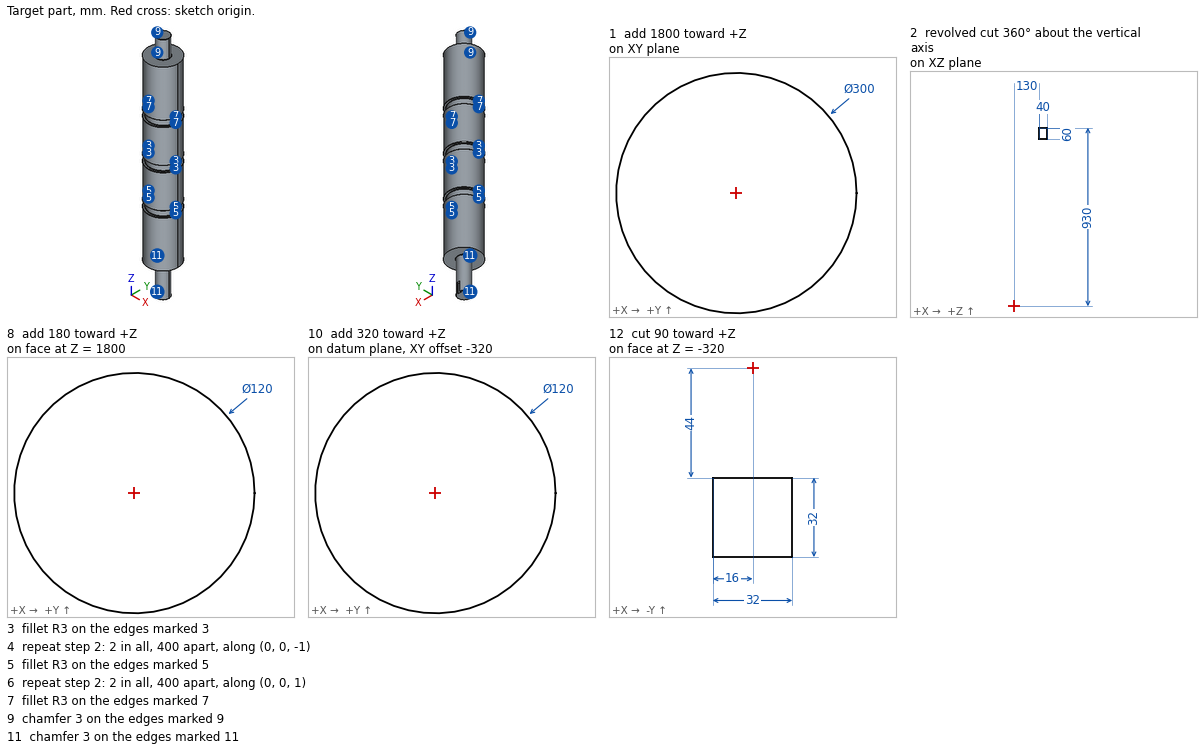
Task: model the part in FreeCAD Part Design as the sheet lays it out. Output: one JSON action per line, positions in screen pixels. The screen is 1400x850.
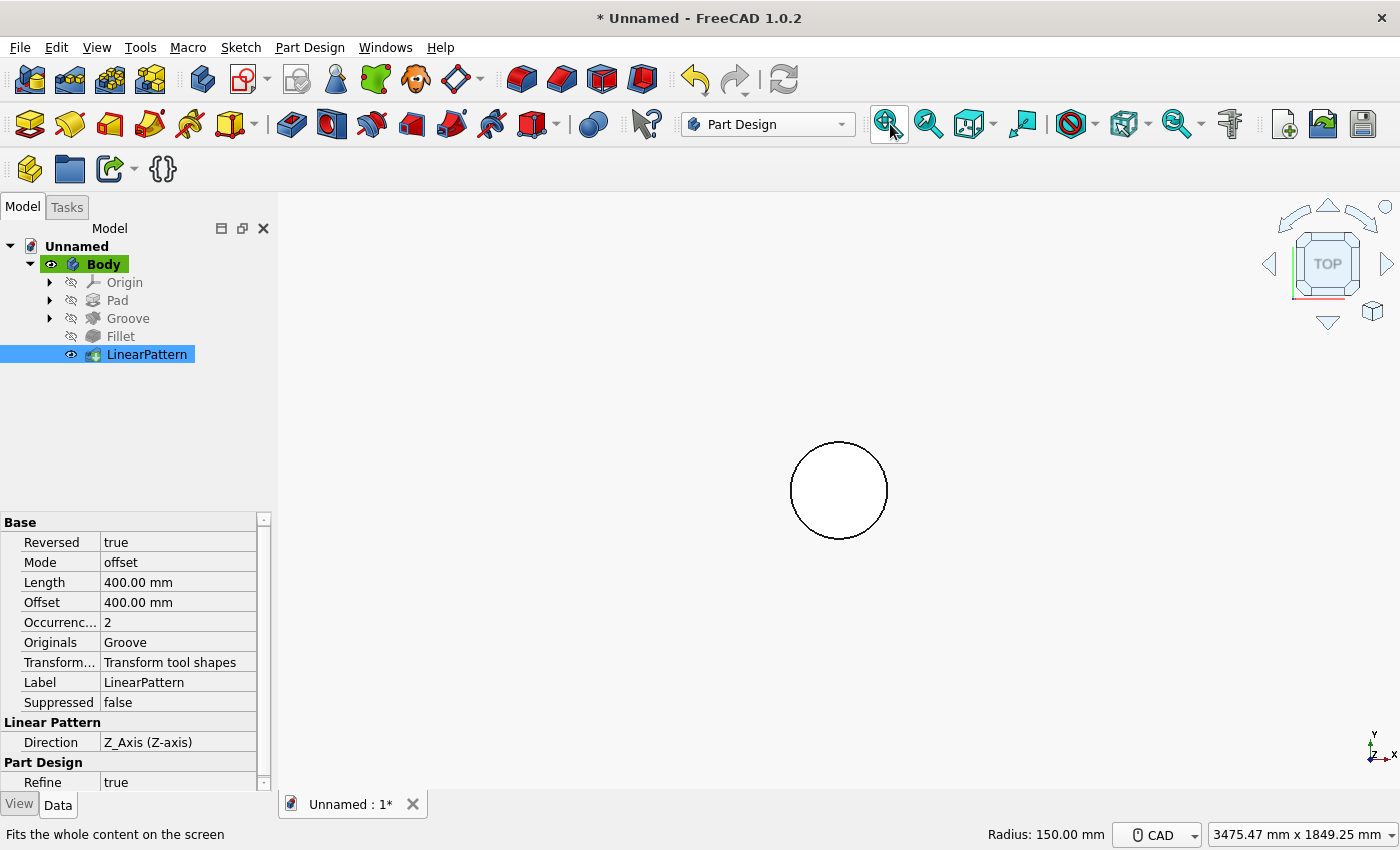
{"action": "key", "text": "0"}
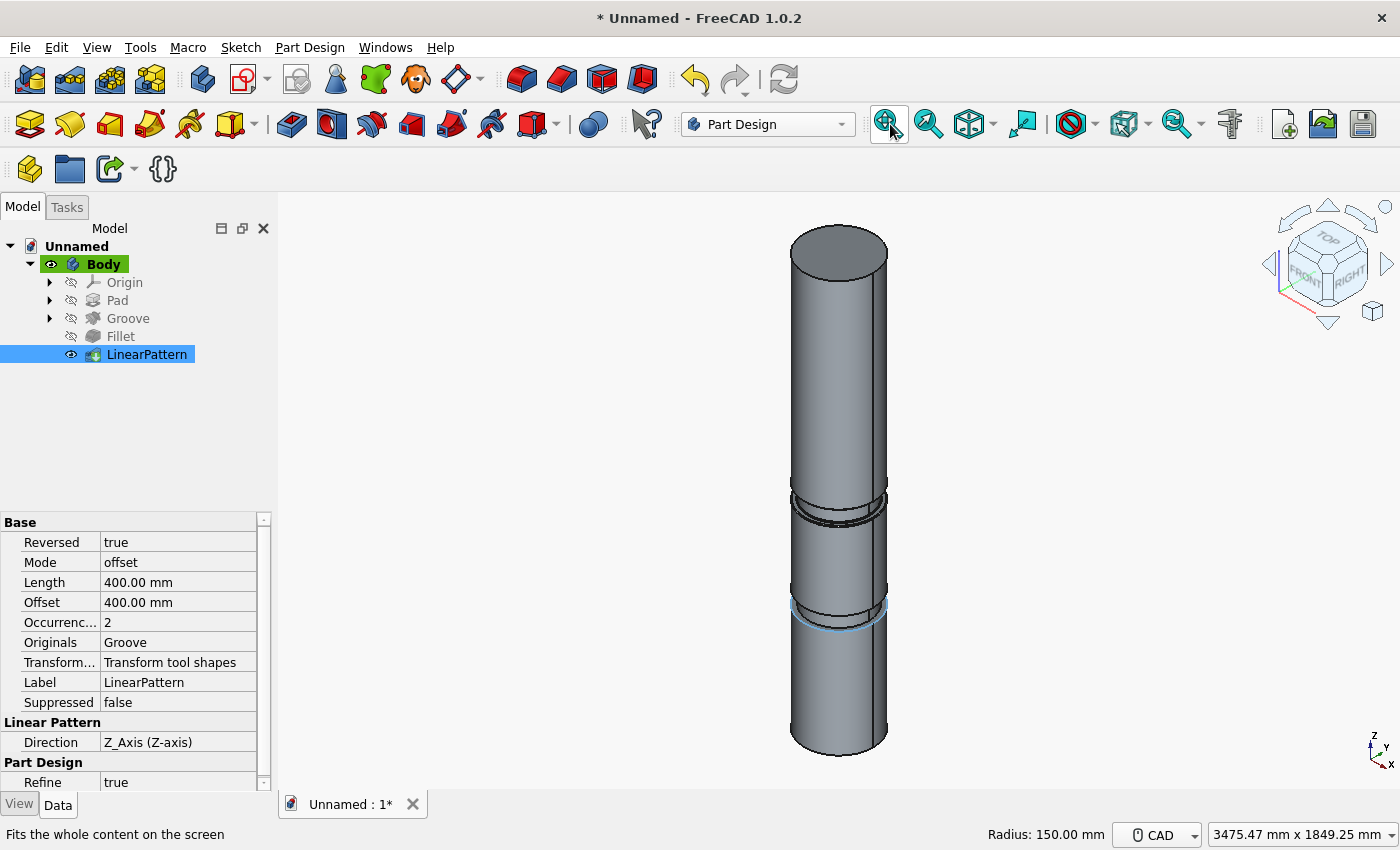
{"action": "key", "text": "1"}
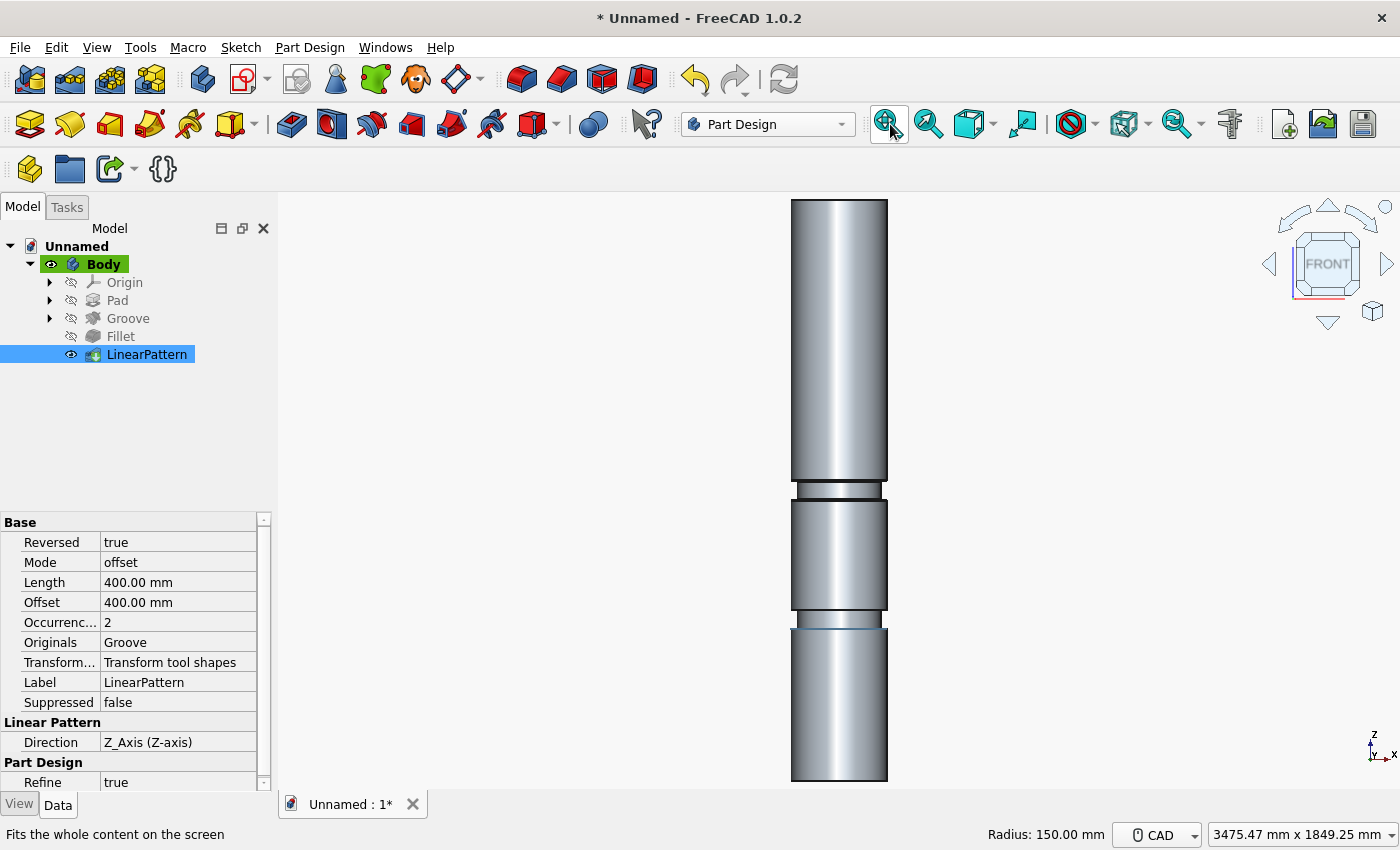
{"action": "left_click", "coordinate": [791, 609], "text": "ctrl"}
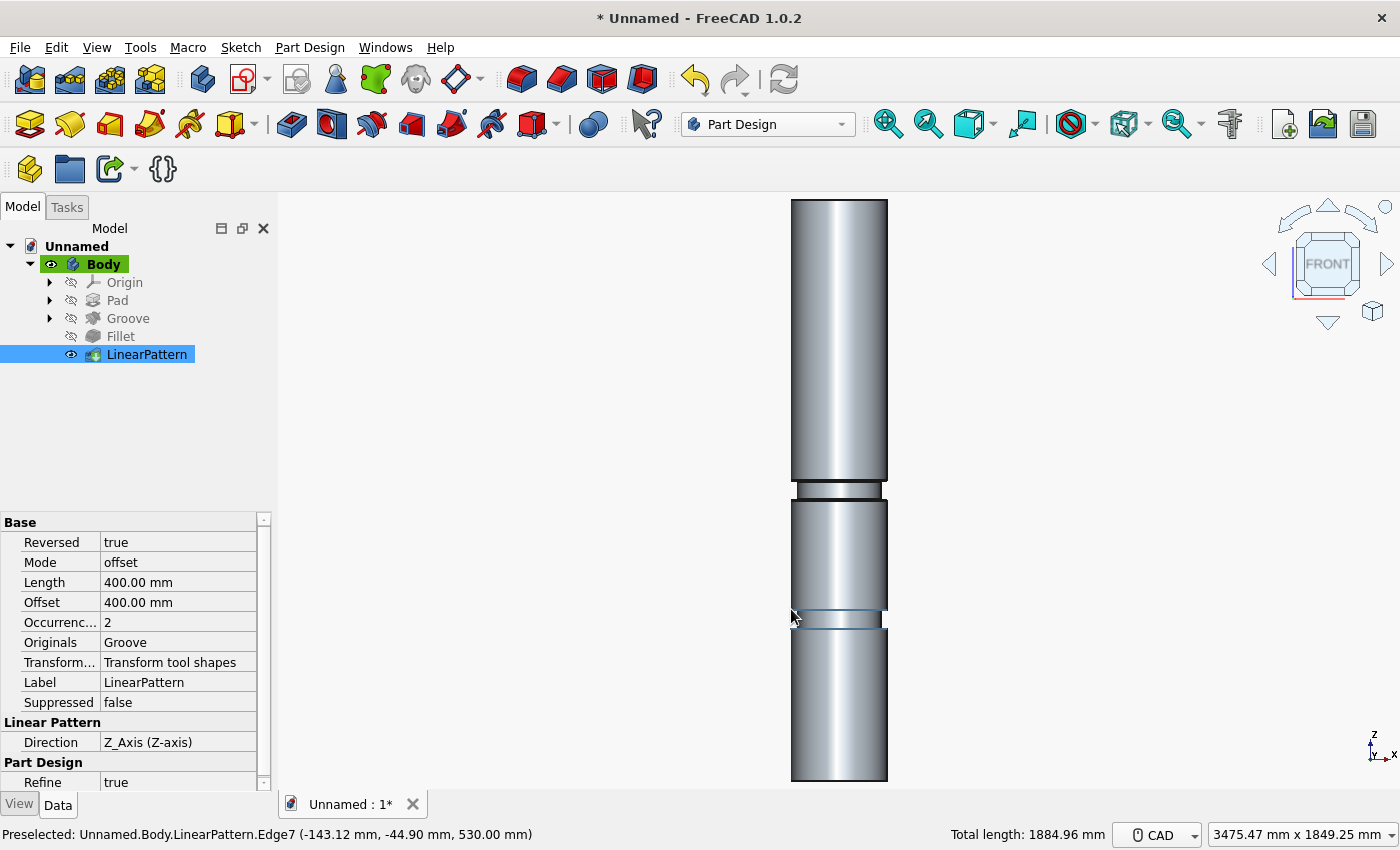
{"action": "key", "text": "3"}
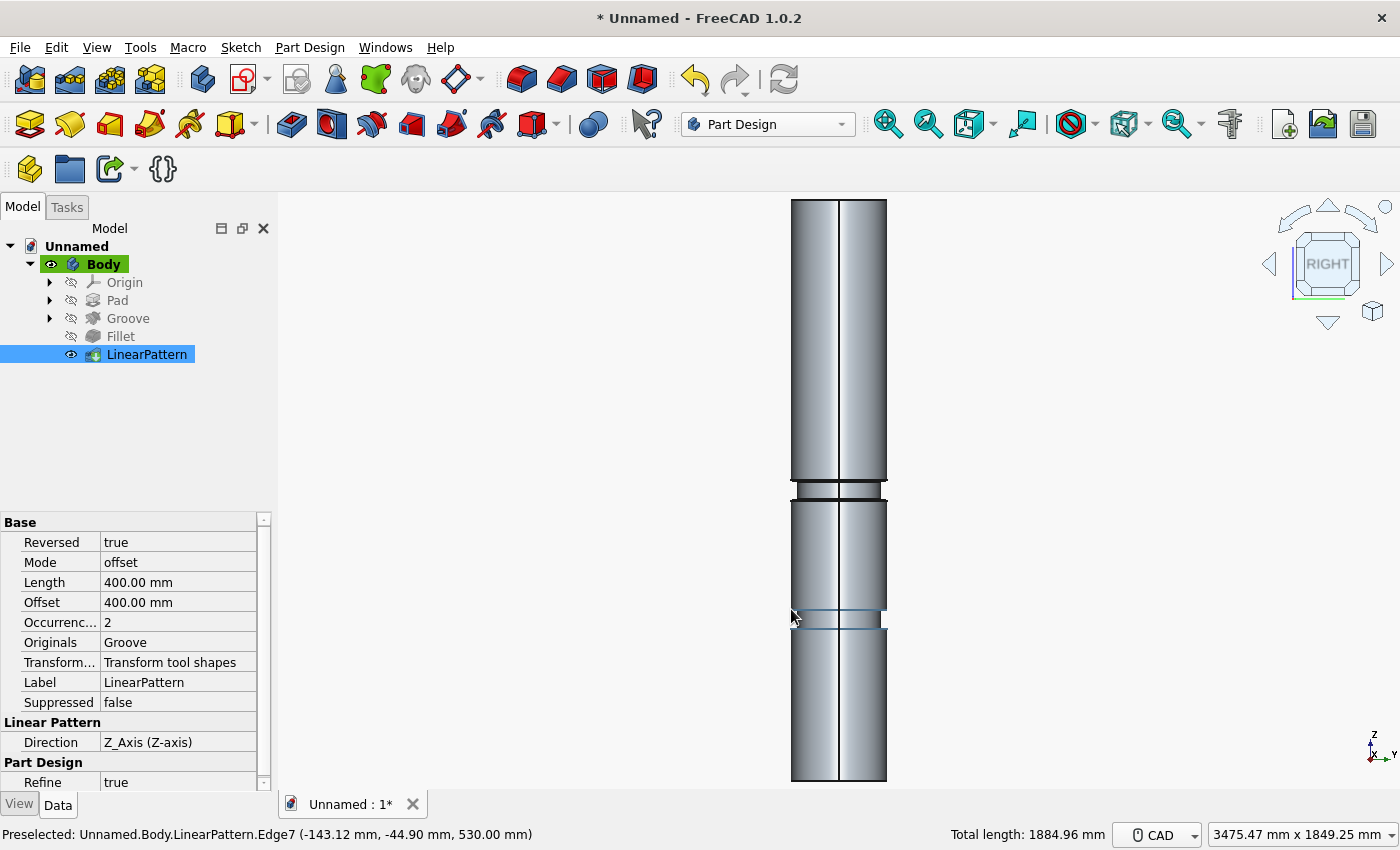
{"action": "key", "text": "5"}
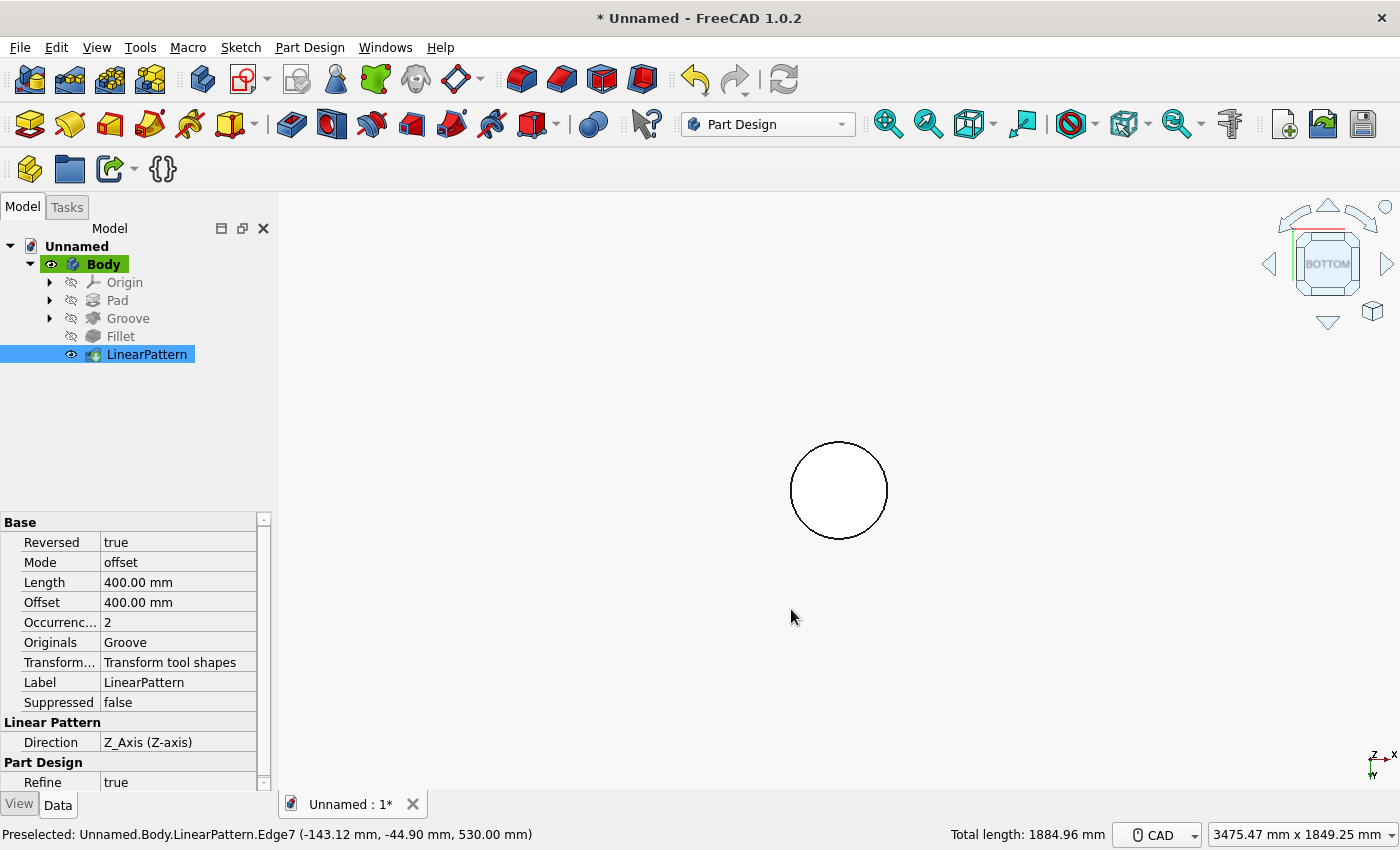
{"action": "left_click", "coordinate": [890, 124]}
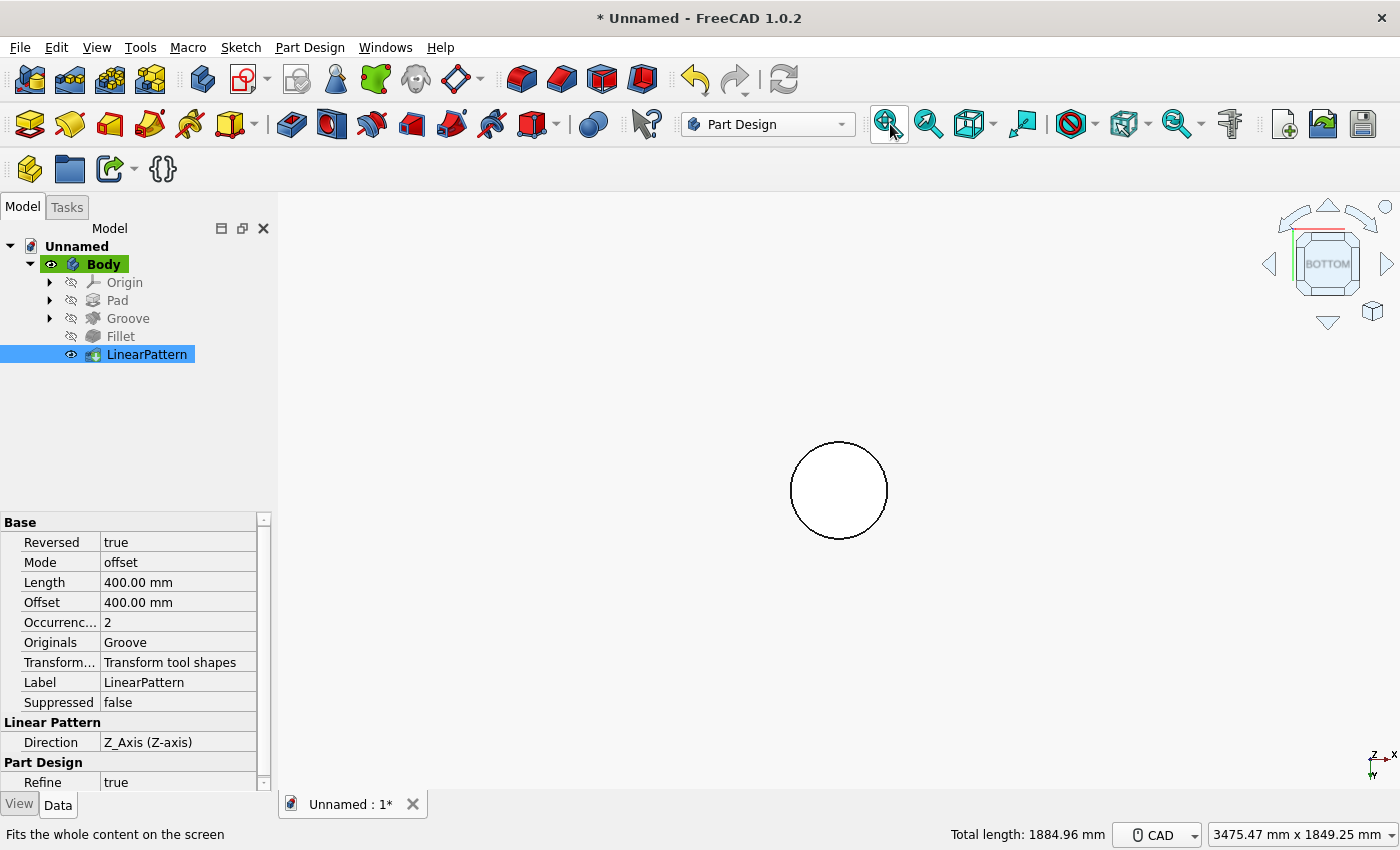
{"action": "key", "text": "4"}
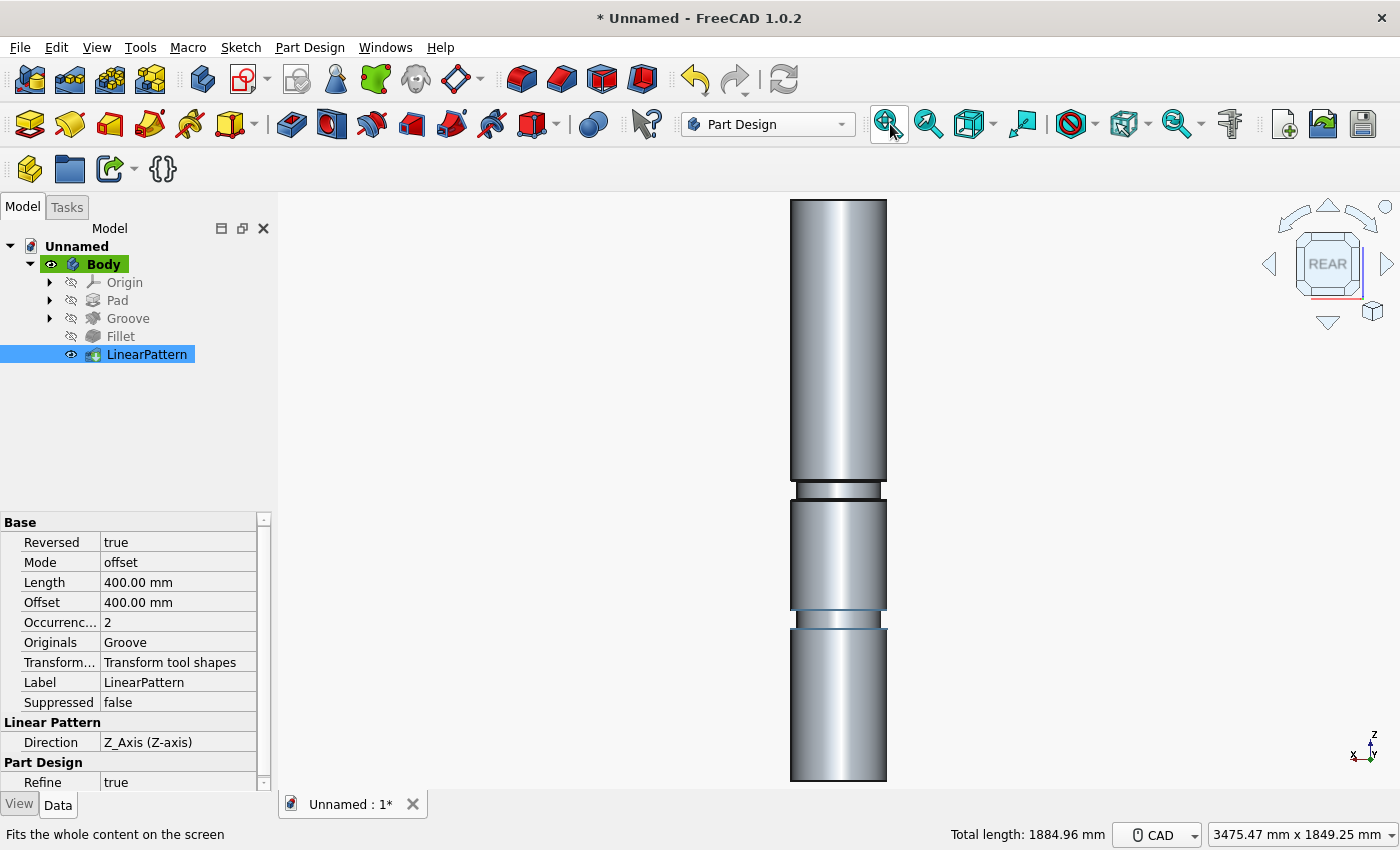
{"action": "key", "text": "6"}